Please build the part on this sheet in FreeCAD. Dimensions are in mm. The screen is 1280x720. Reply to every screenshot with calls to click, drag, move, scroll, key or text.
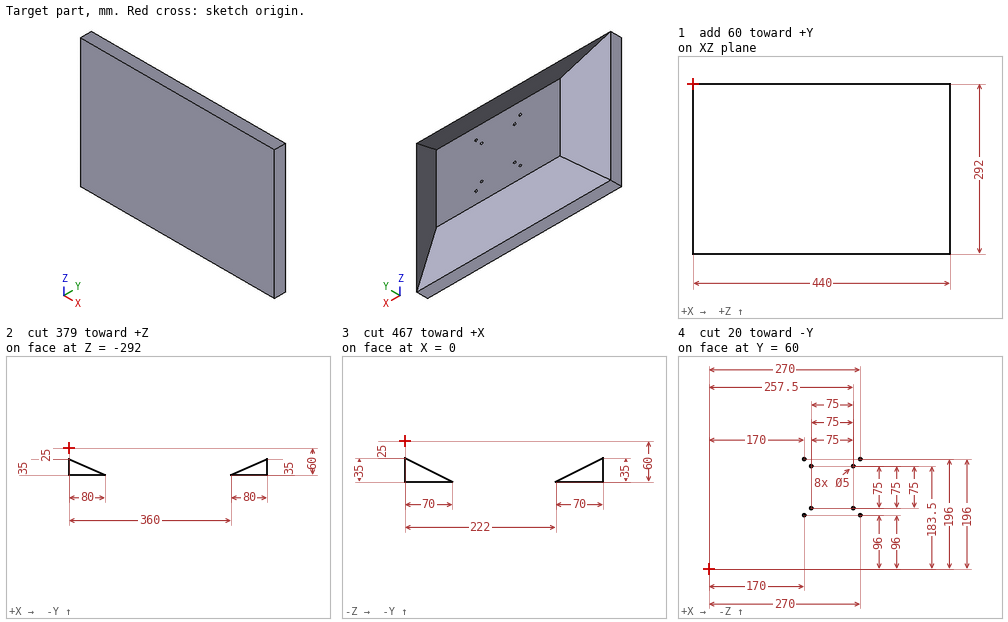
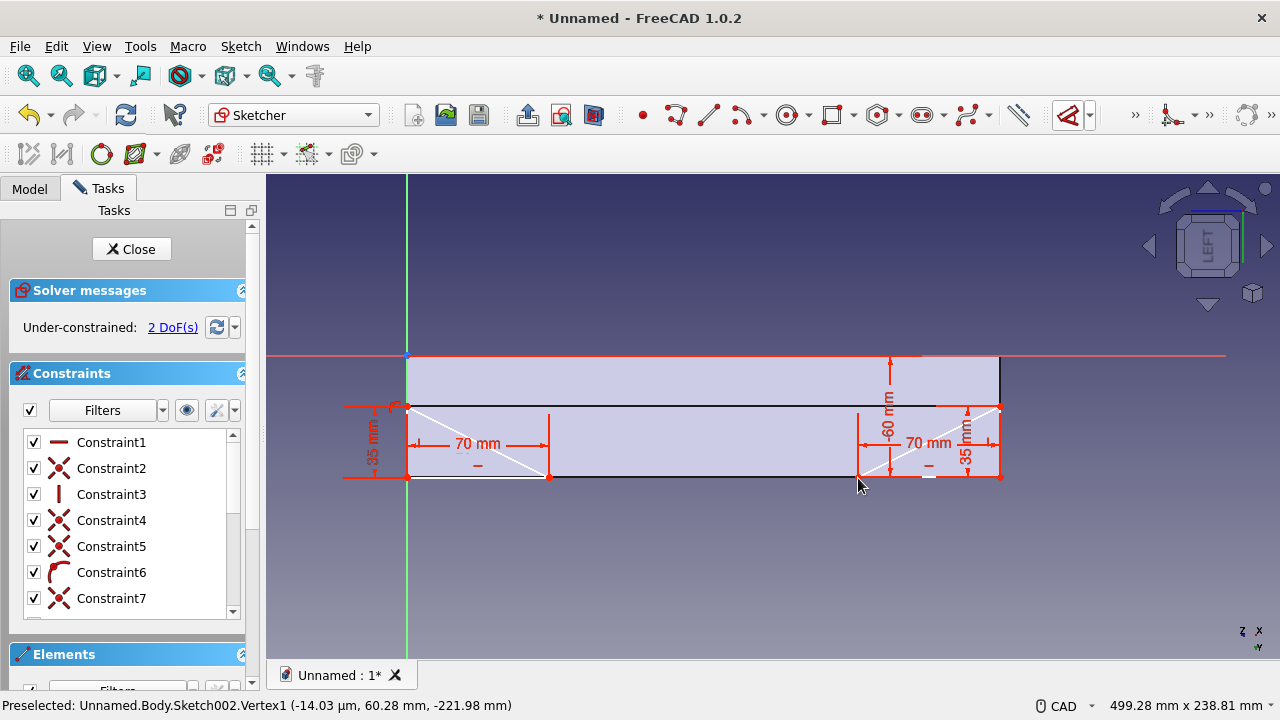
click(407, 407)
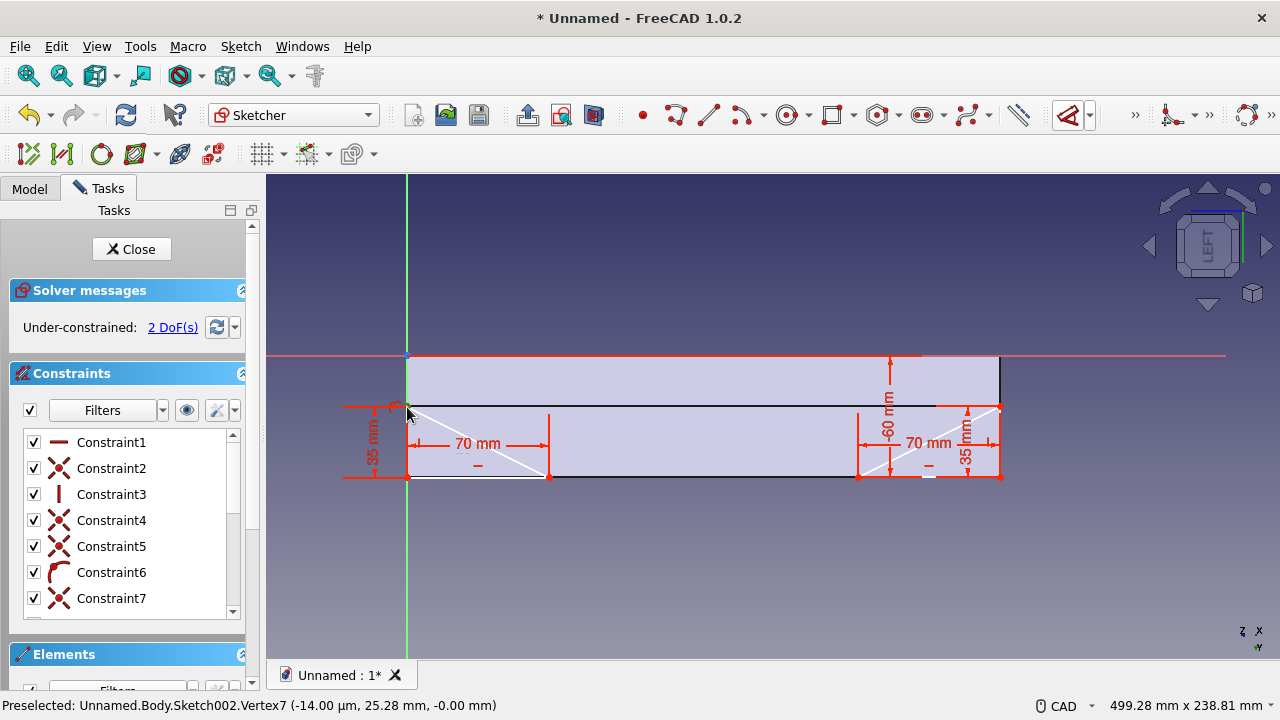
key(i)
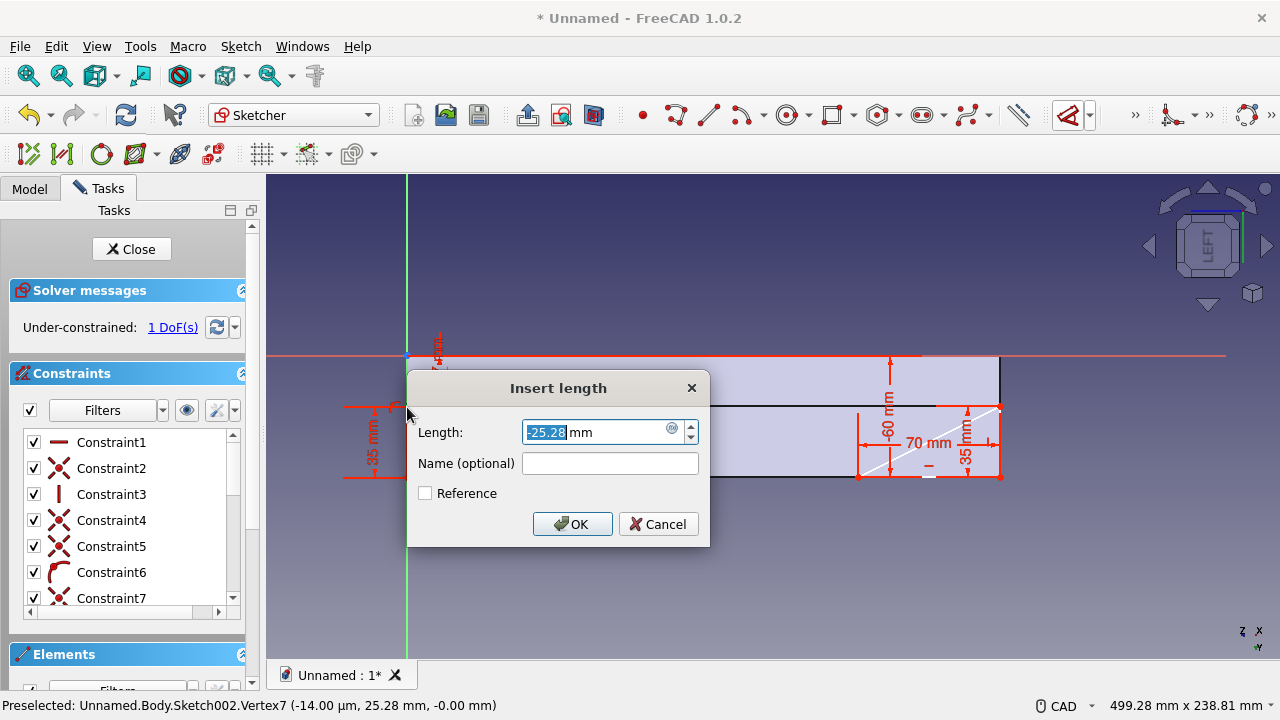
text(-25)
key(Return)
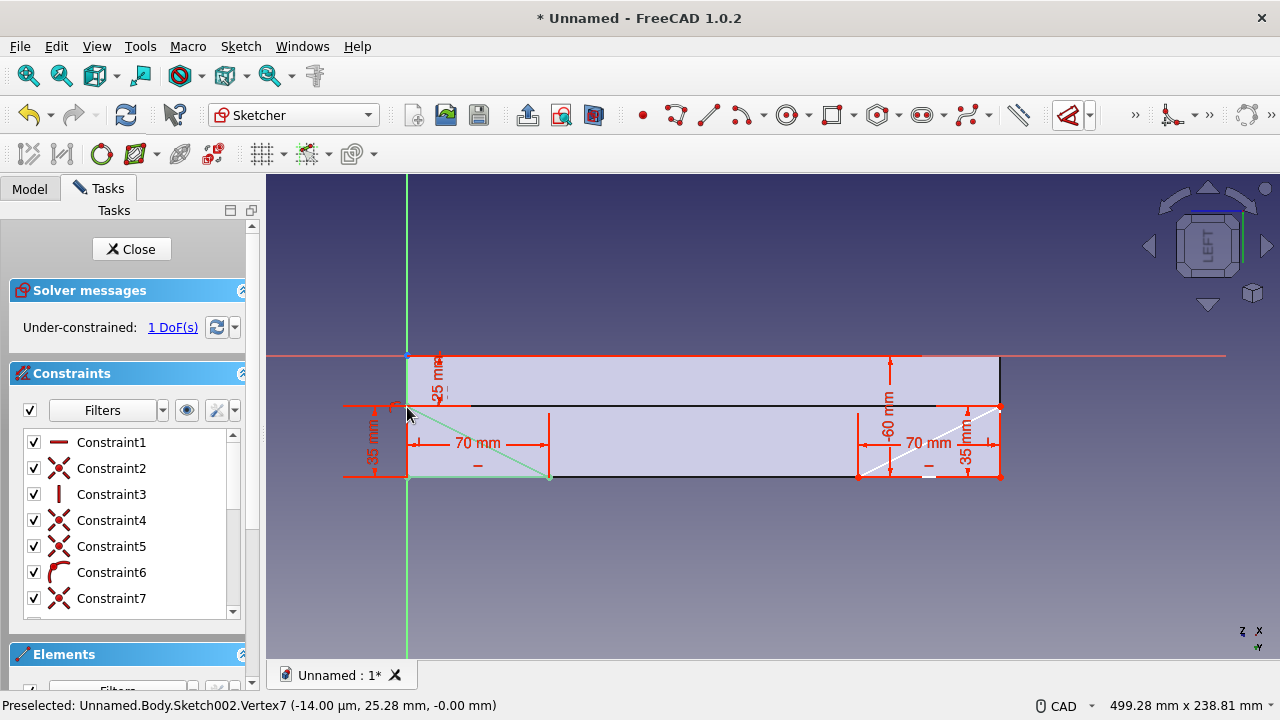
click(858, 477)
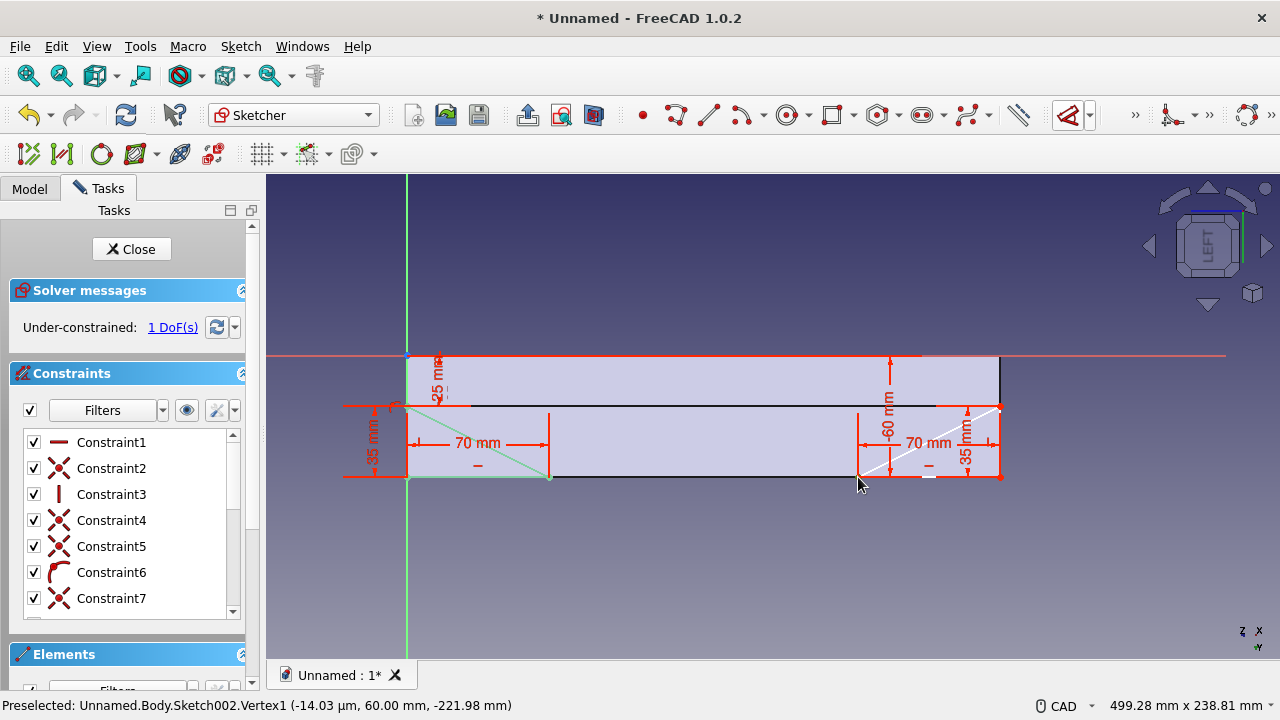
key(l)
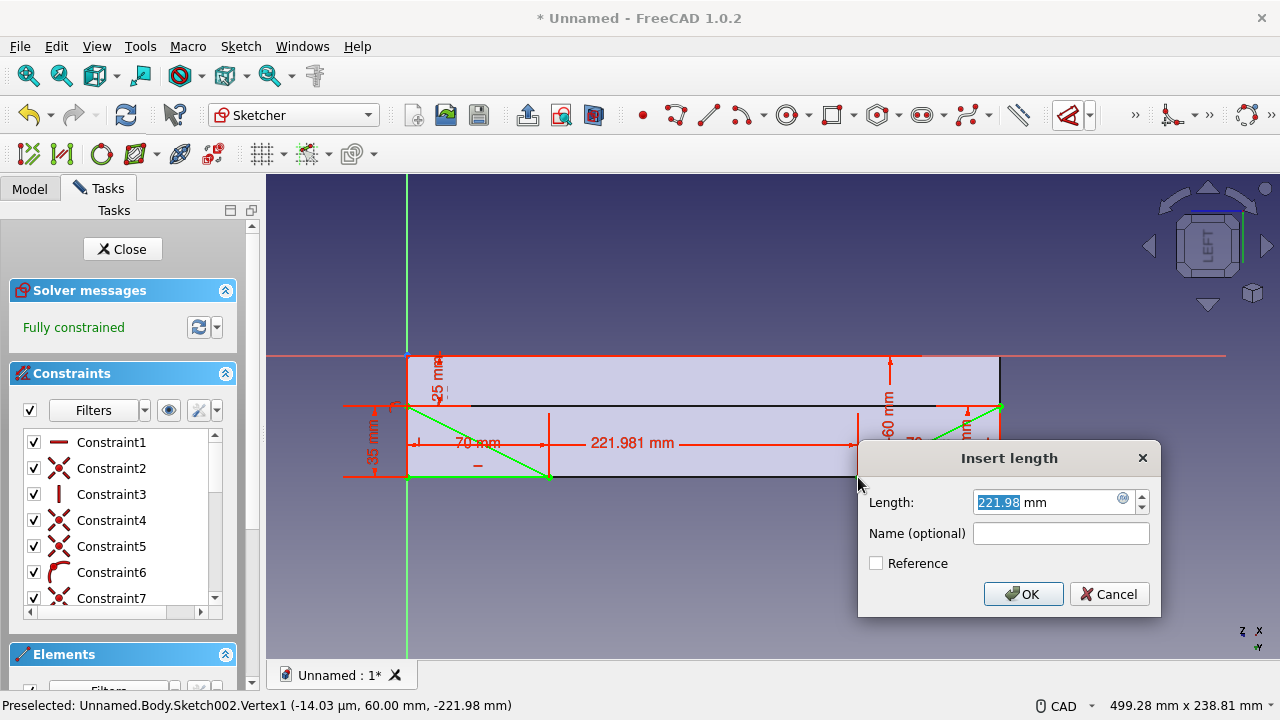
text(222)
key(Return)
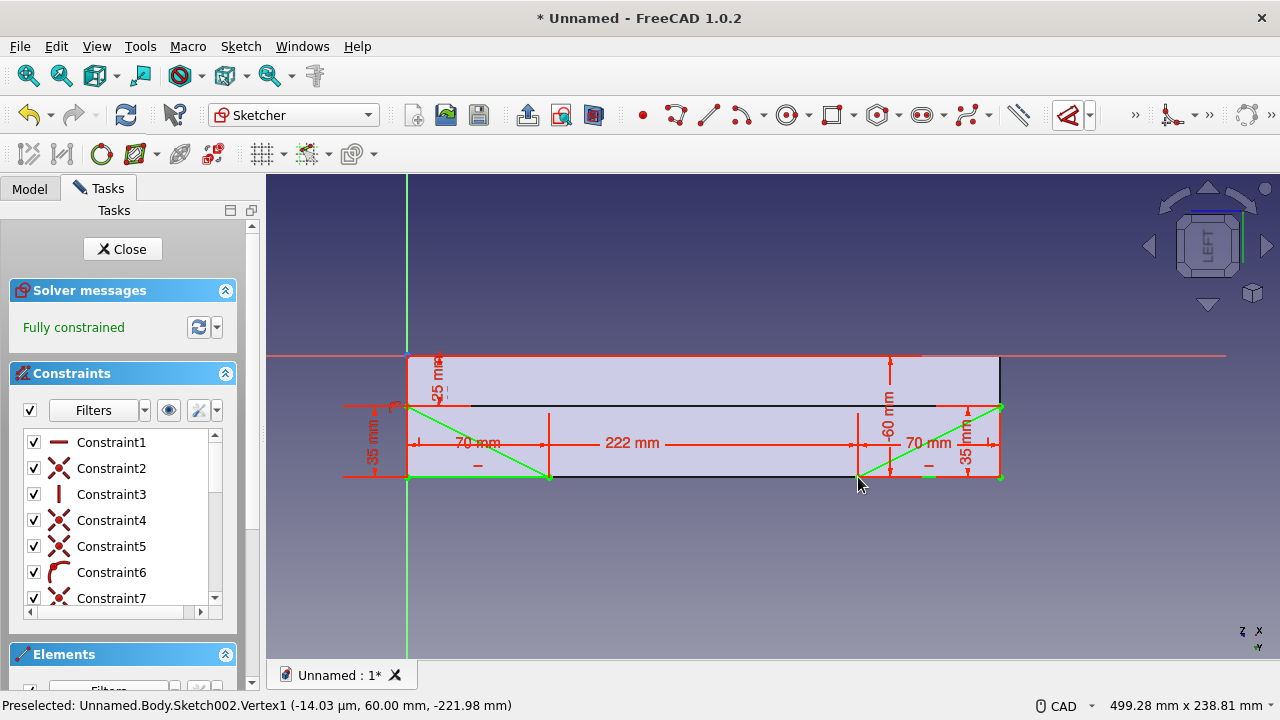
click(123, 249)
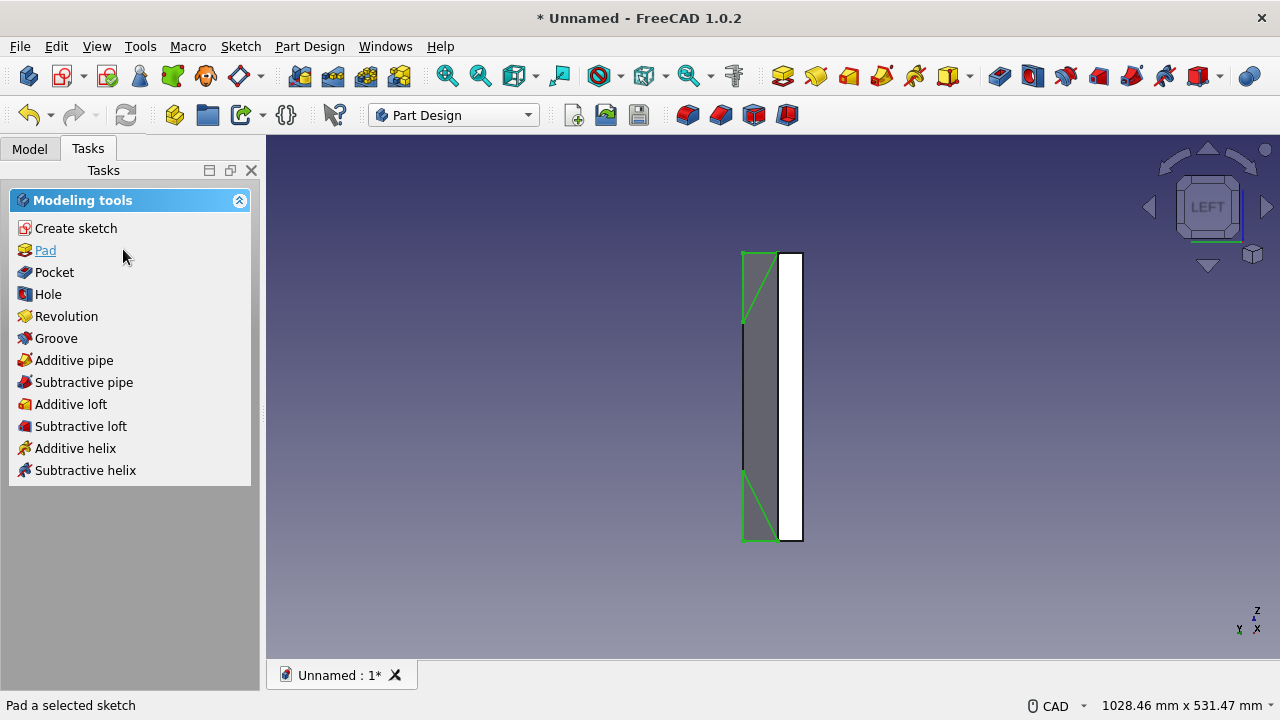
click(1000, 76)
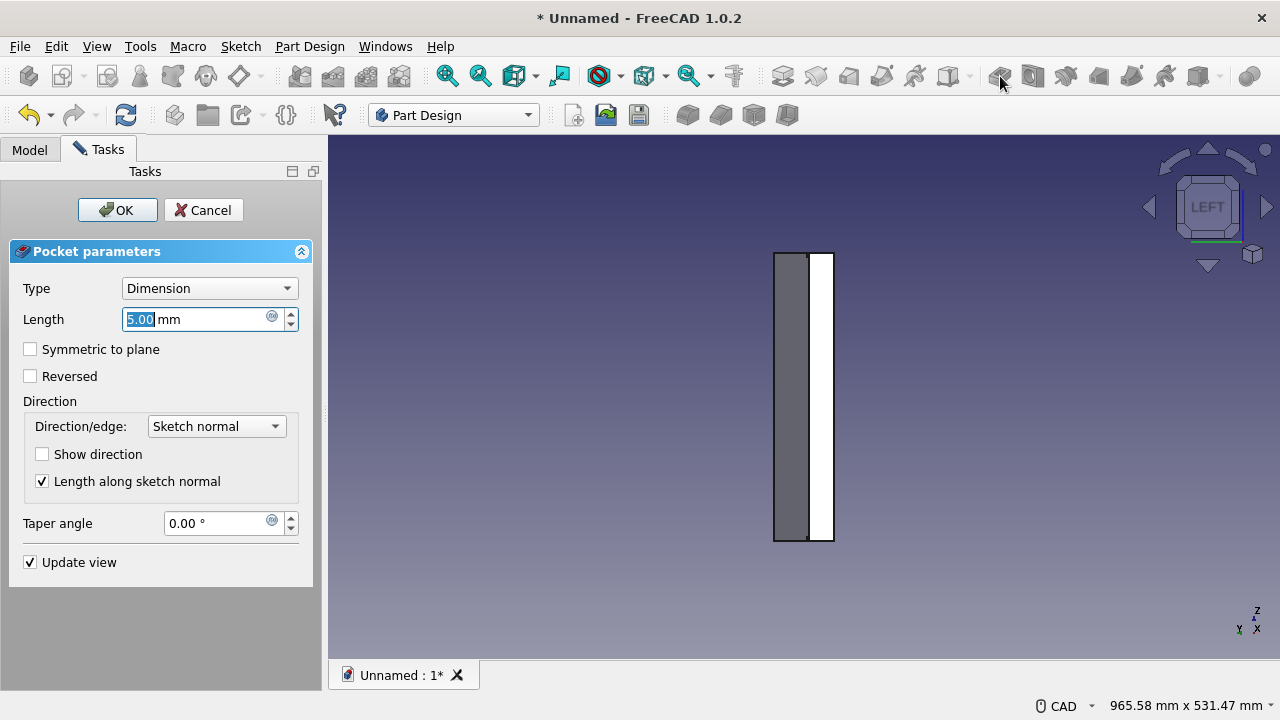
text(467)
key(Tab)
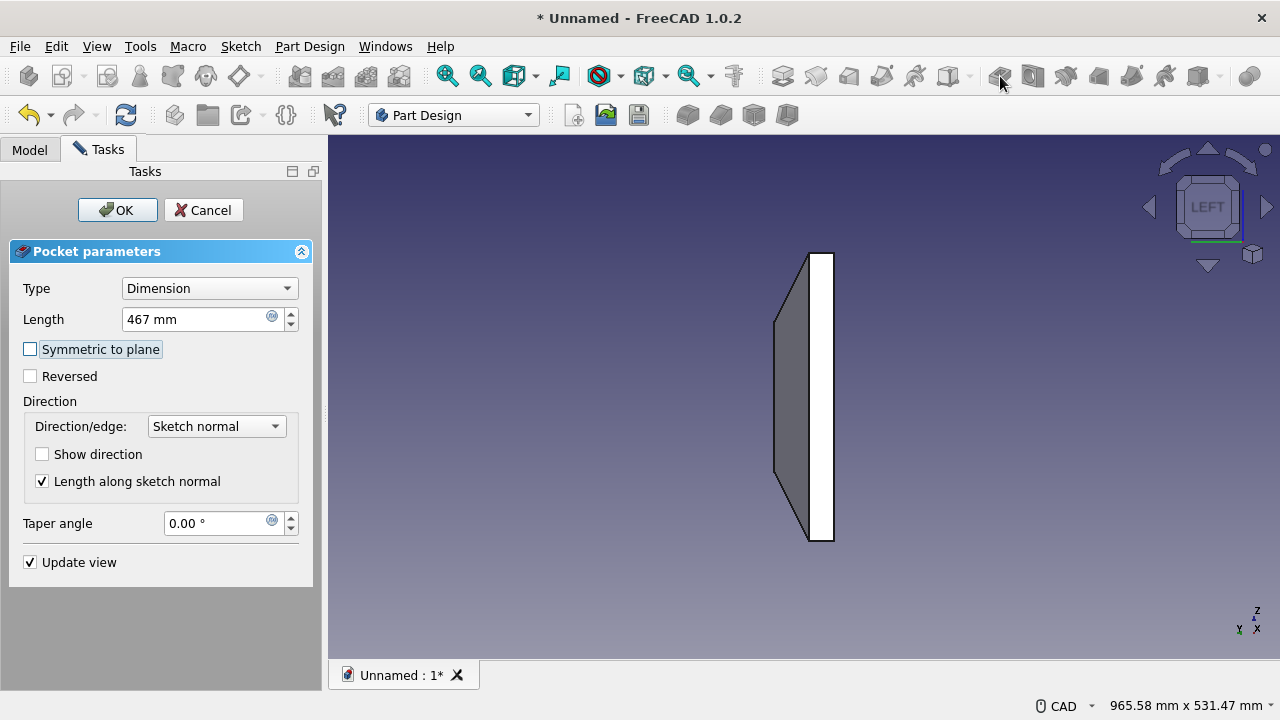
click(118, 210)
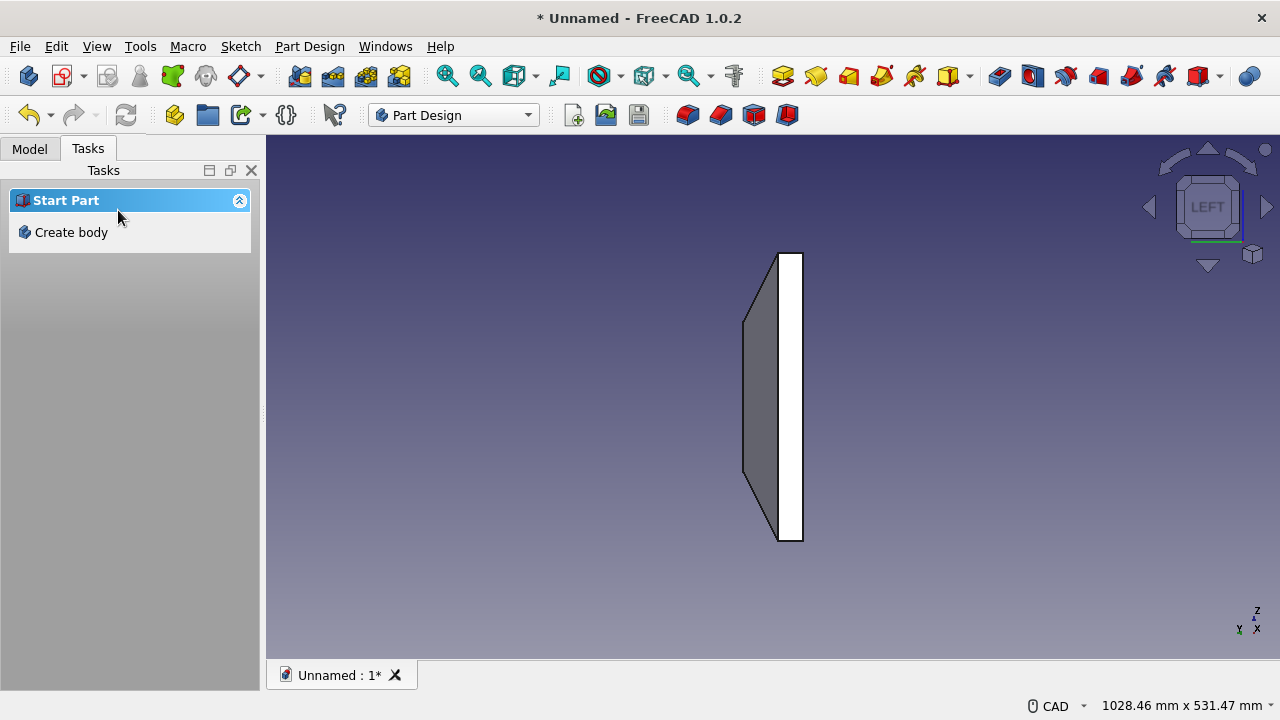
key(4)